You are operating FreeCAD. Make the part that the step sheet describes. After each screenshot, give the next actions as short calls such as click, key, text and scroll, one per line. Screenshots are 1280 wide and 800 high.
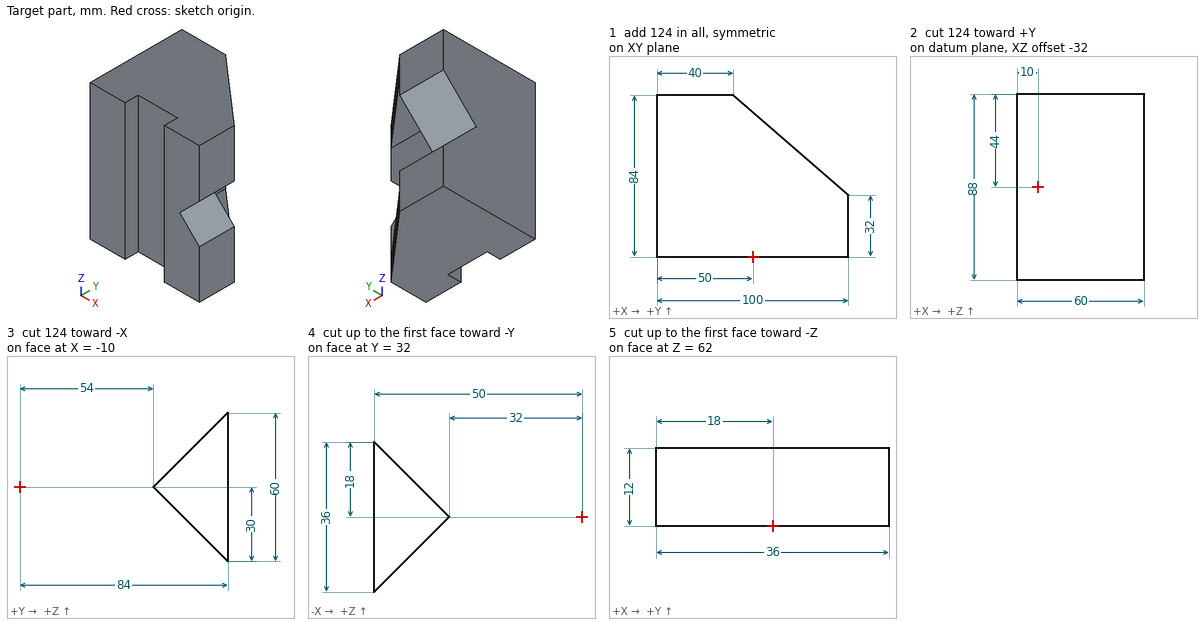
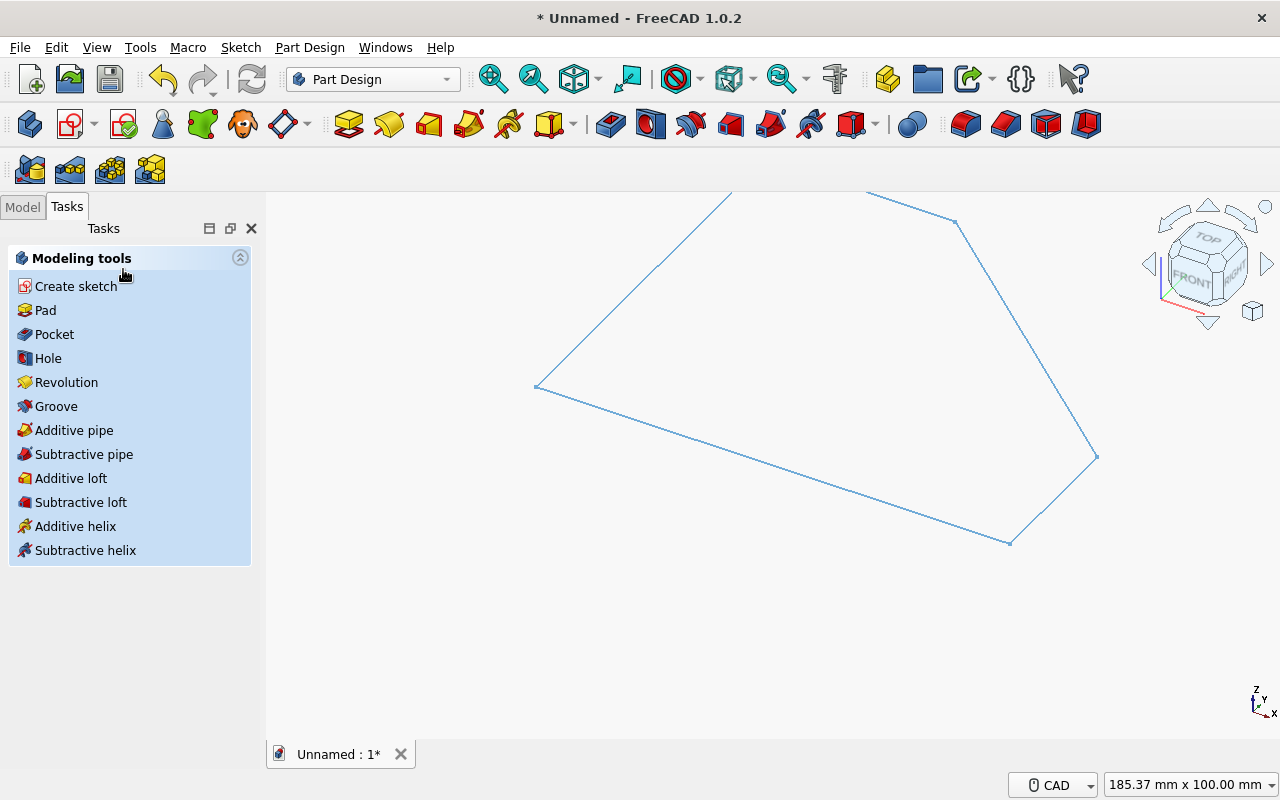
click(350, 124)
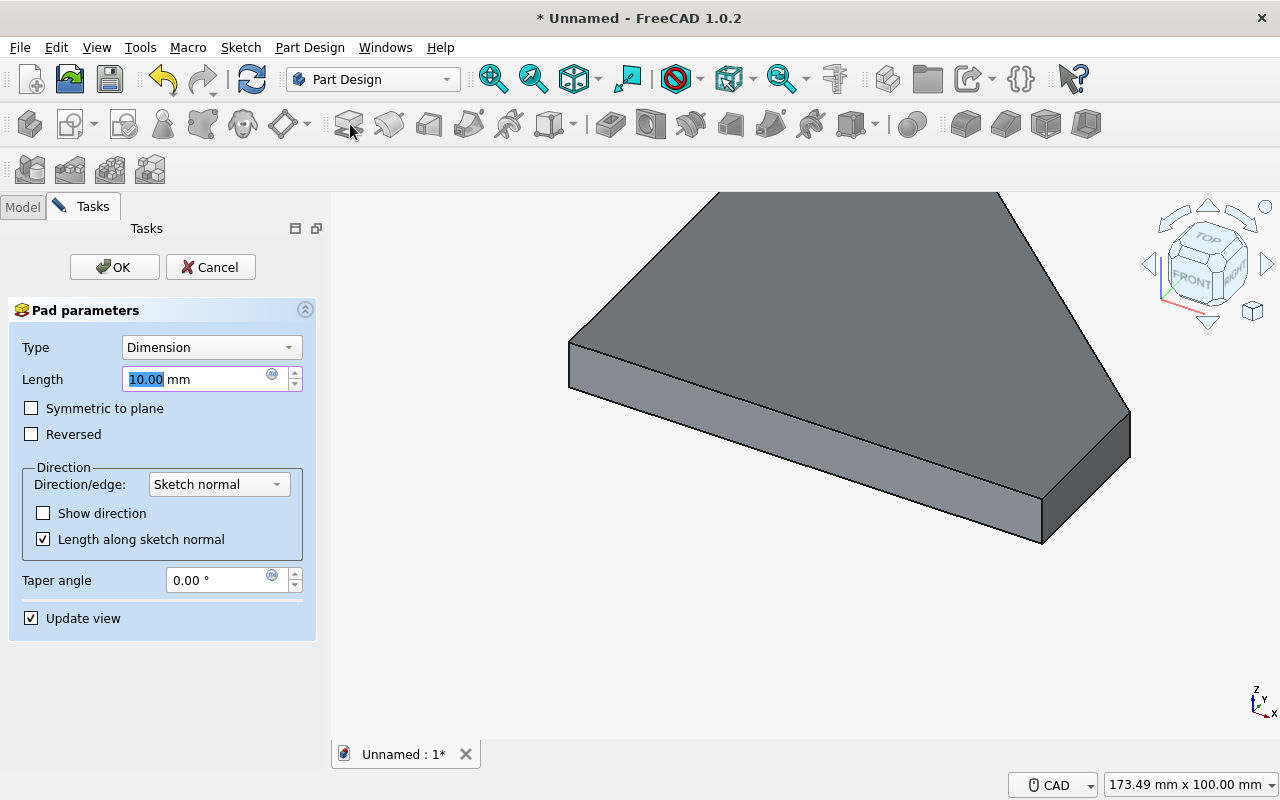
text(124)
key(Tab)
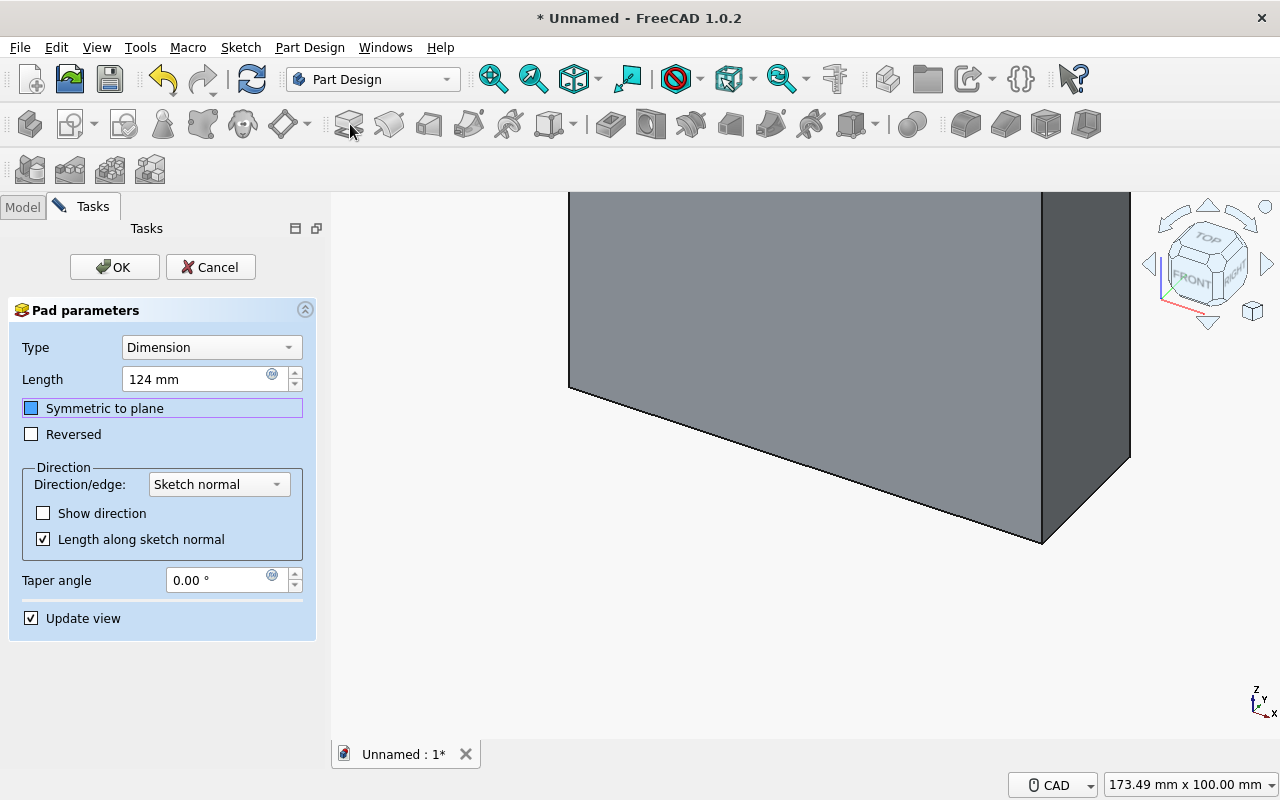
click(30, 408)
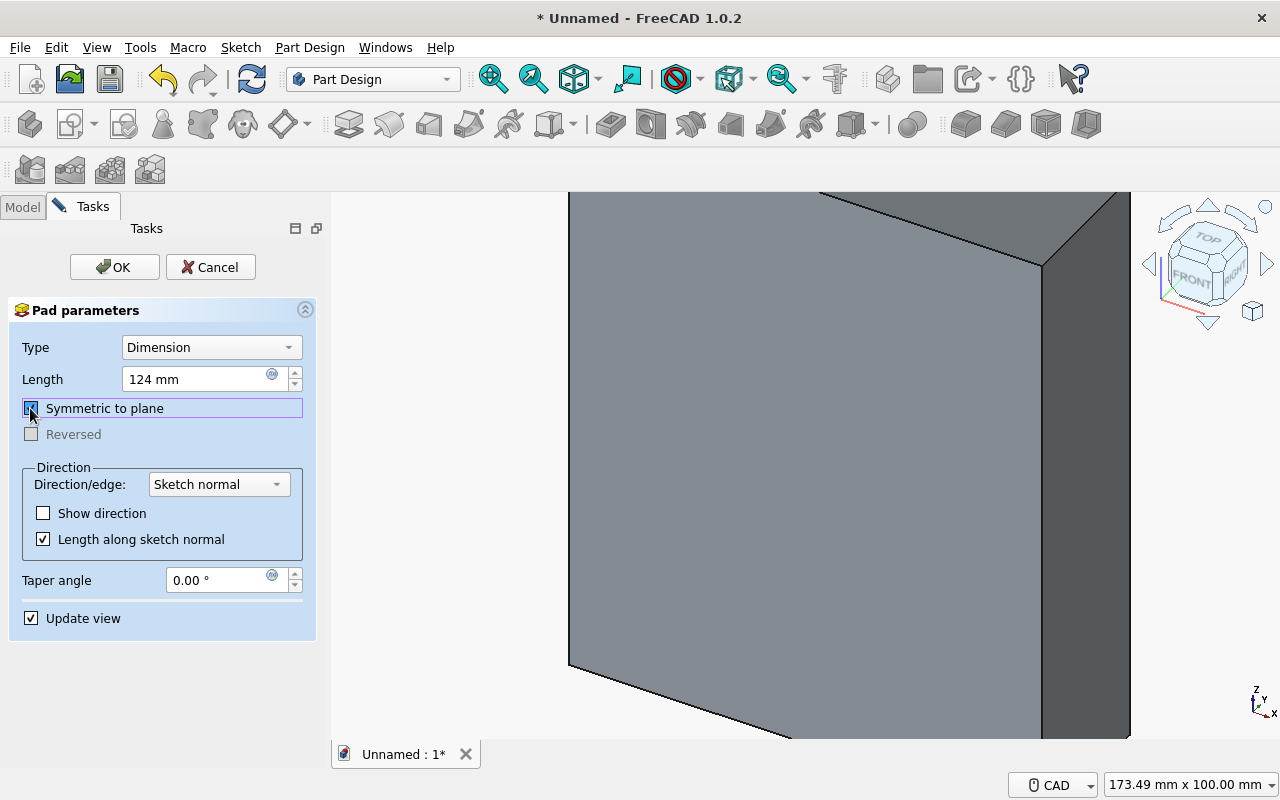
click(115, 267)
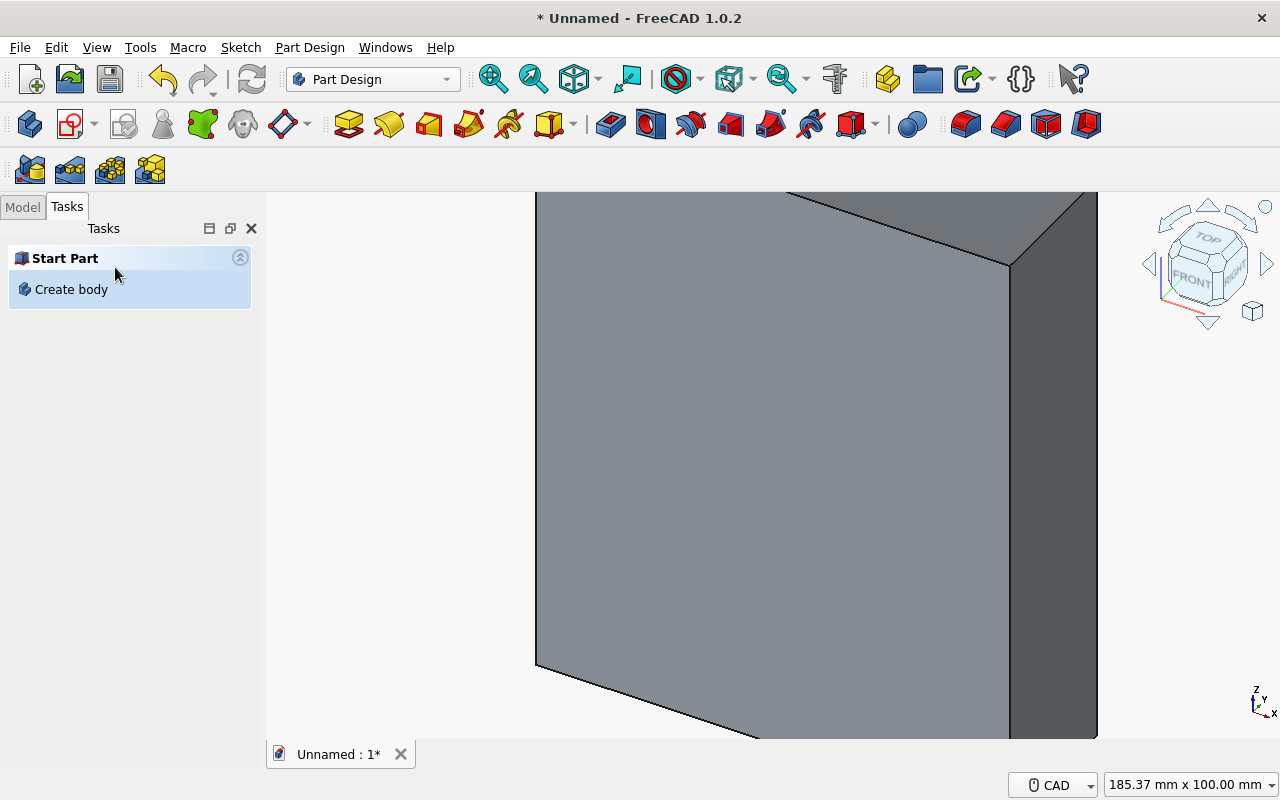
click(494, 80)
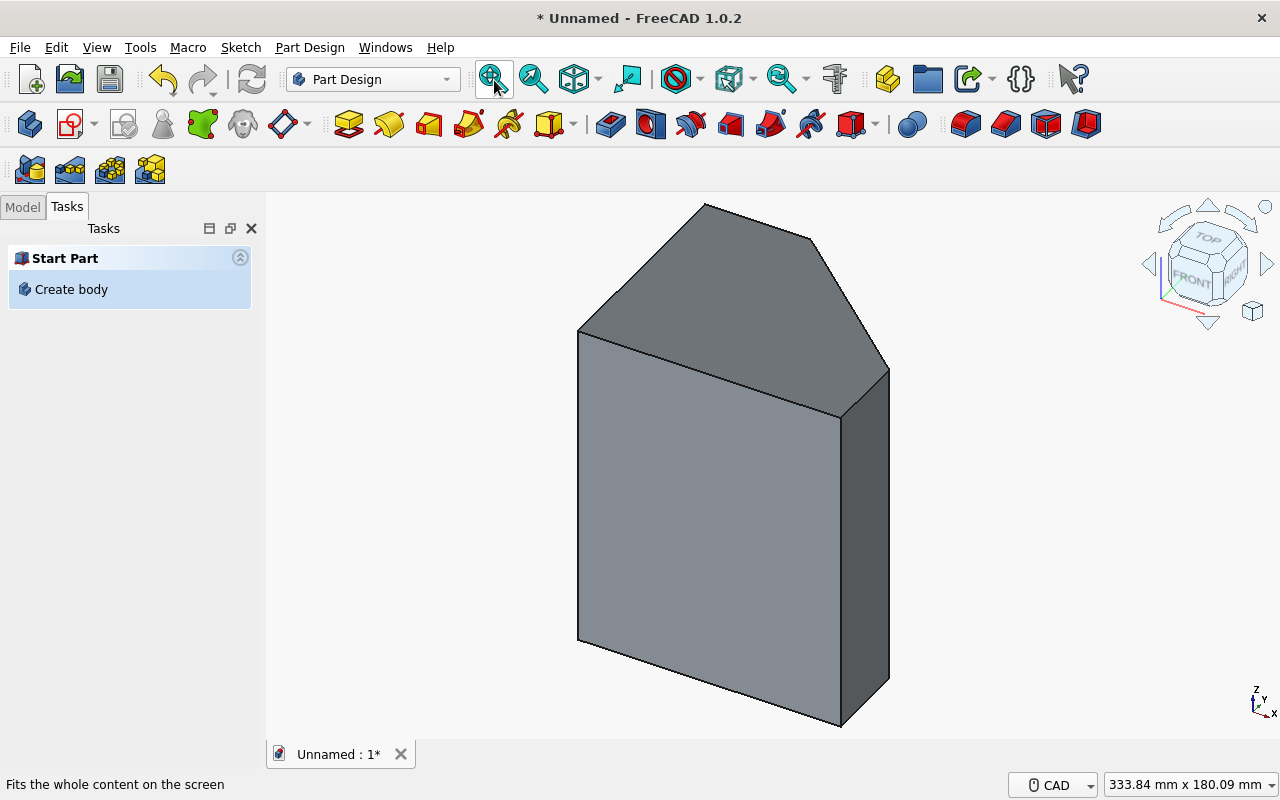
click(23, 206)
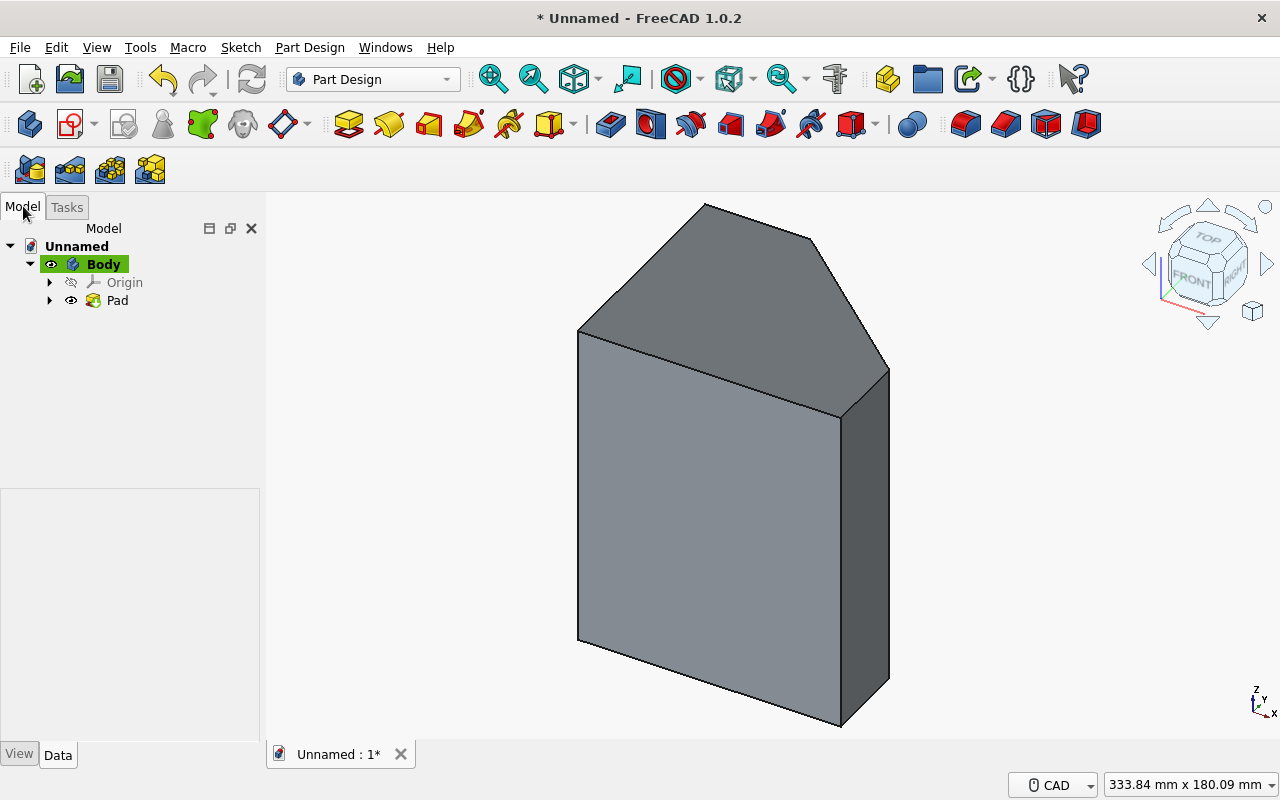
click(50, 282)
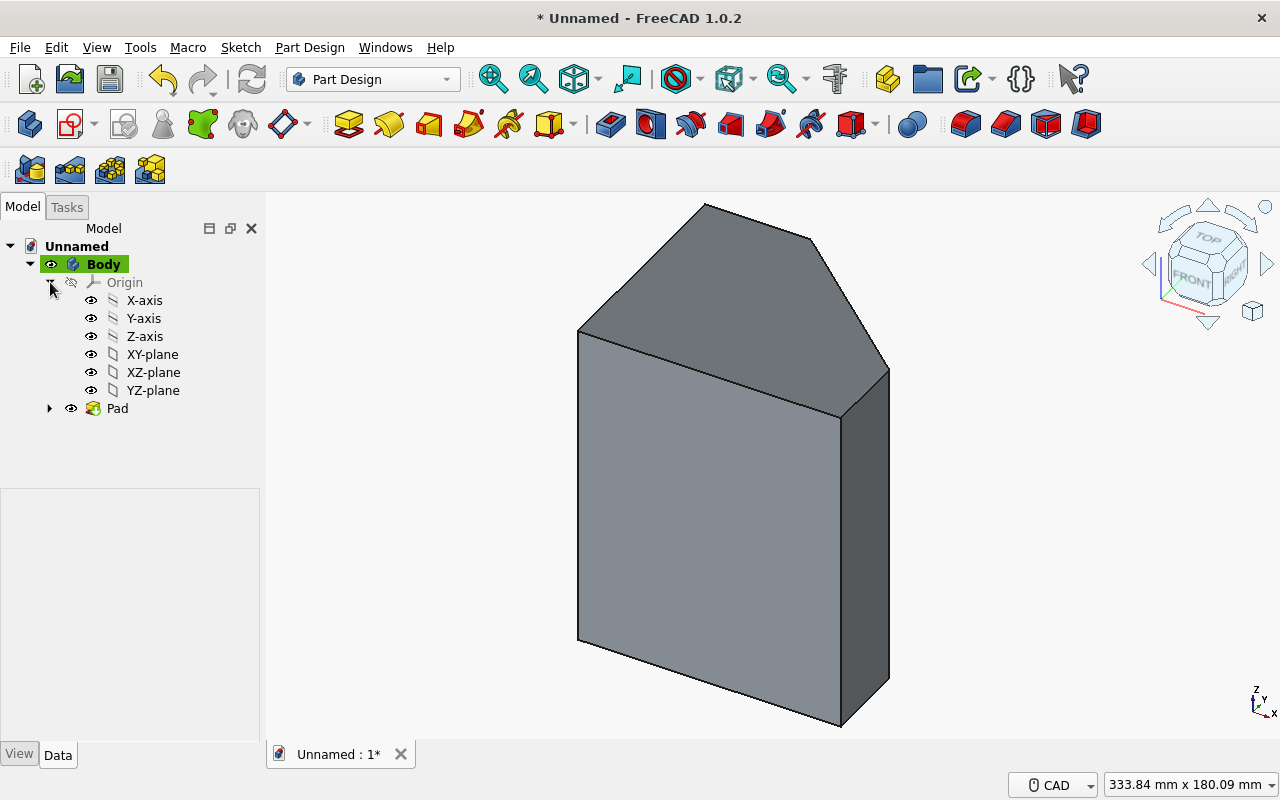
click(136, 372)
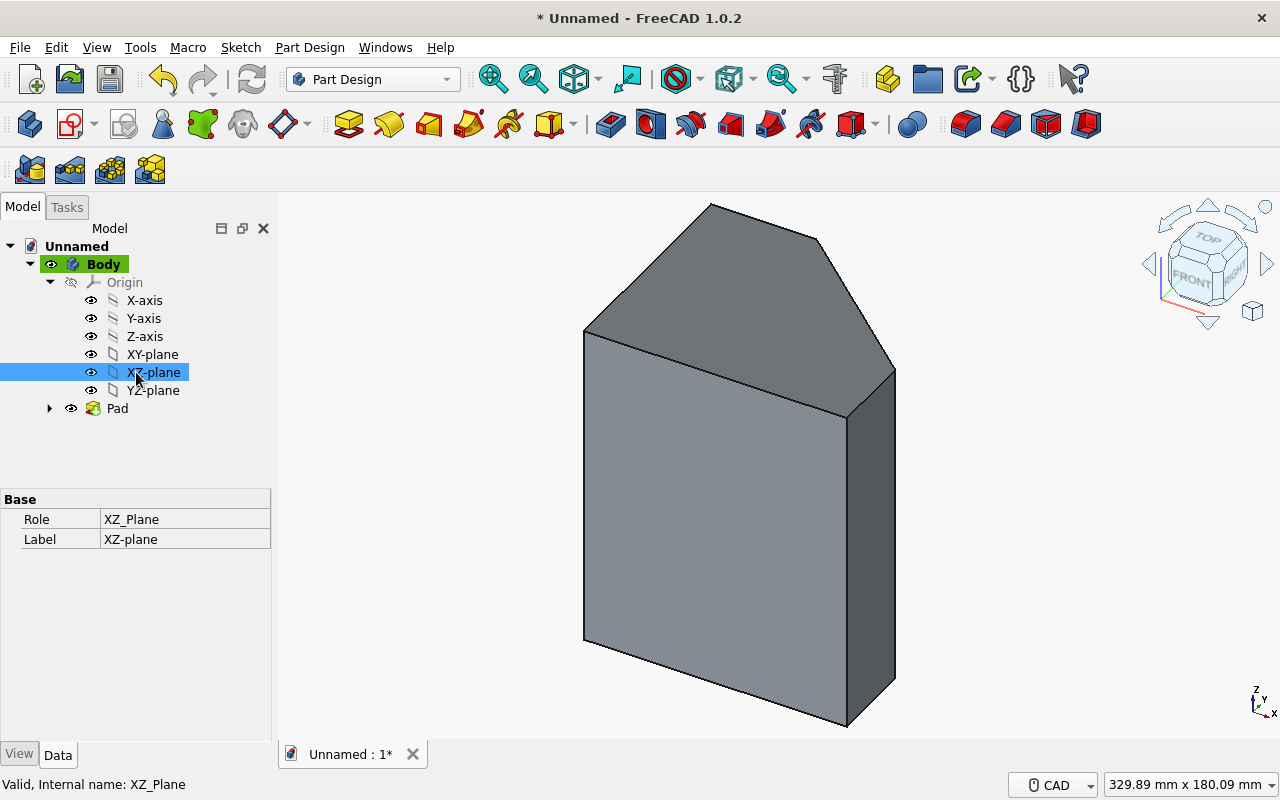
click(284, 124)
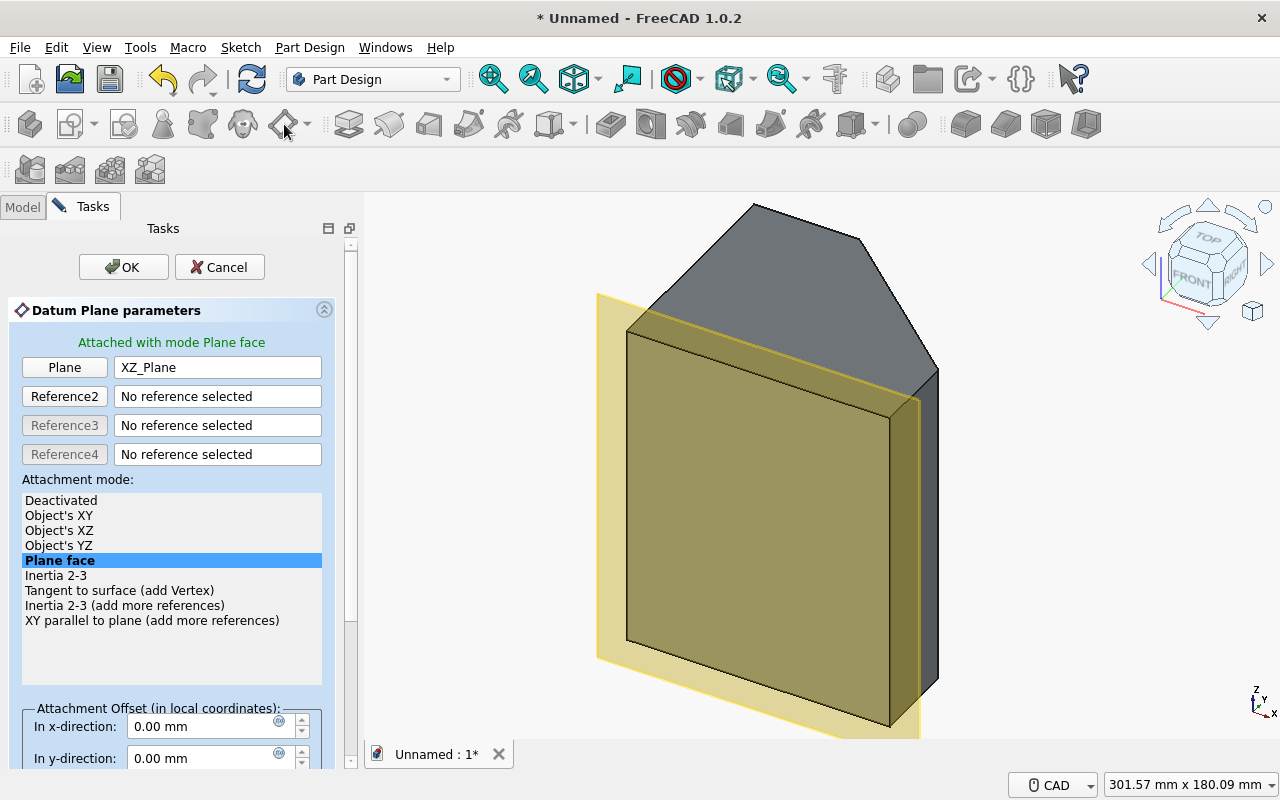
scroll(351, 503, down, 2)